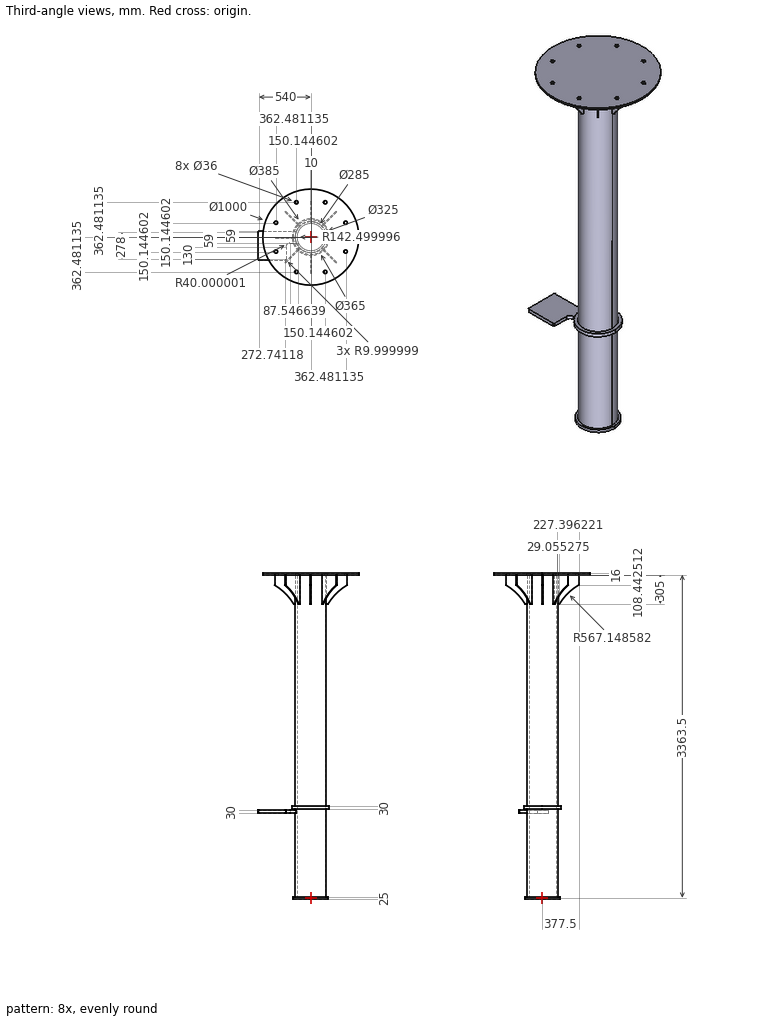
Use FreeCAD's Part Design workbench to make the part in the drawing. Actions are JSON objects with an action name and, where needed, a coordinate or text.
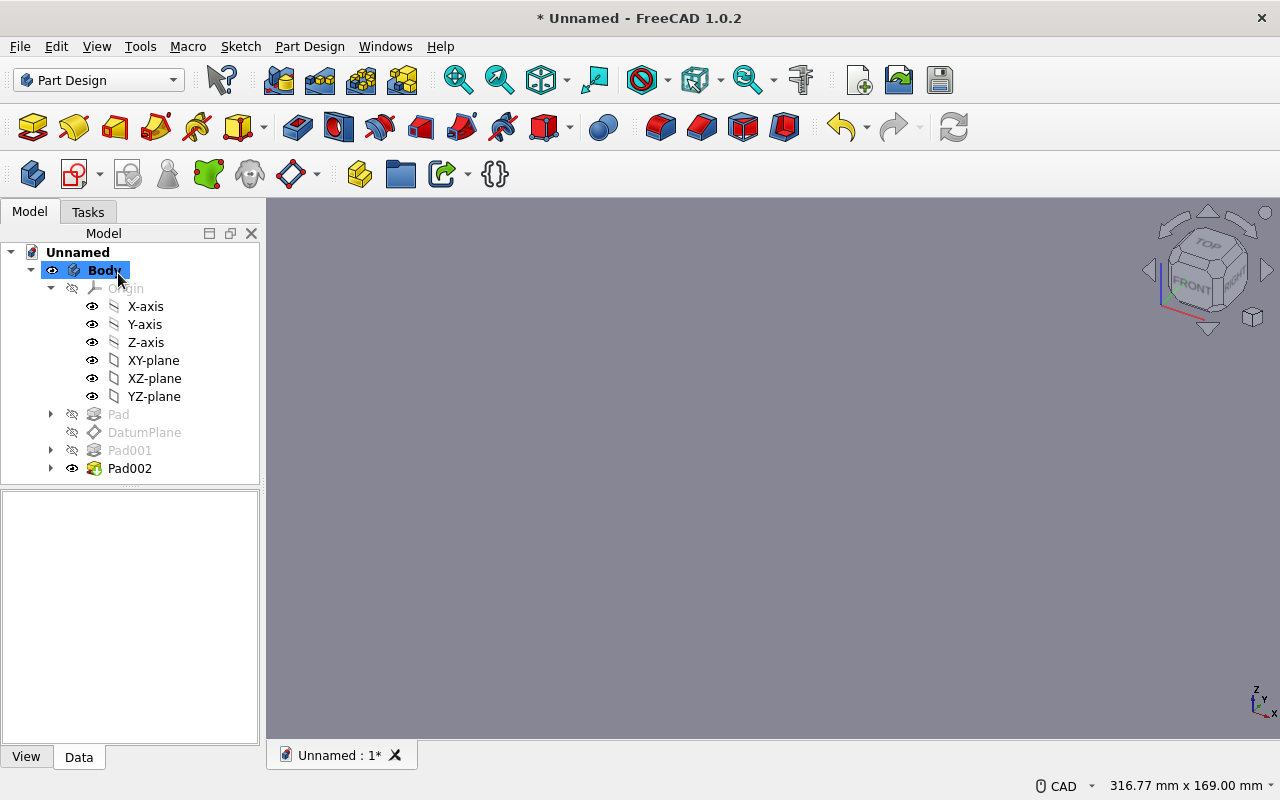
{"action": "key", "text": "v f"}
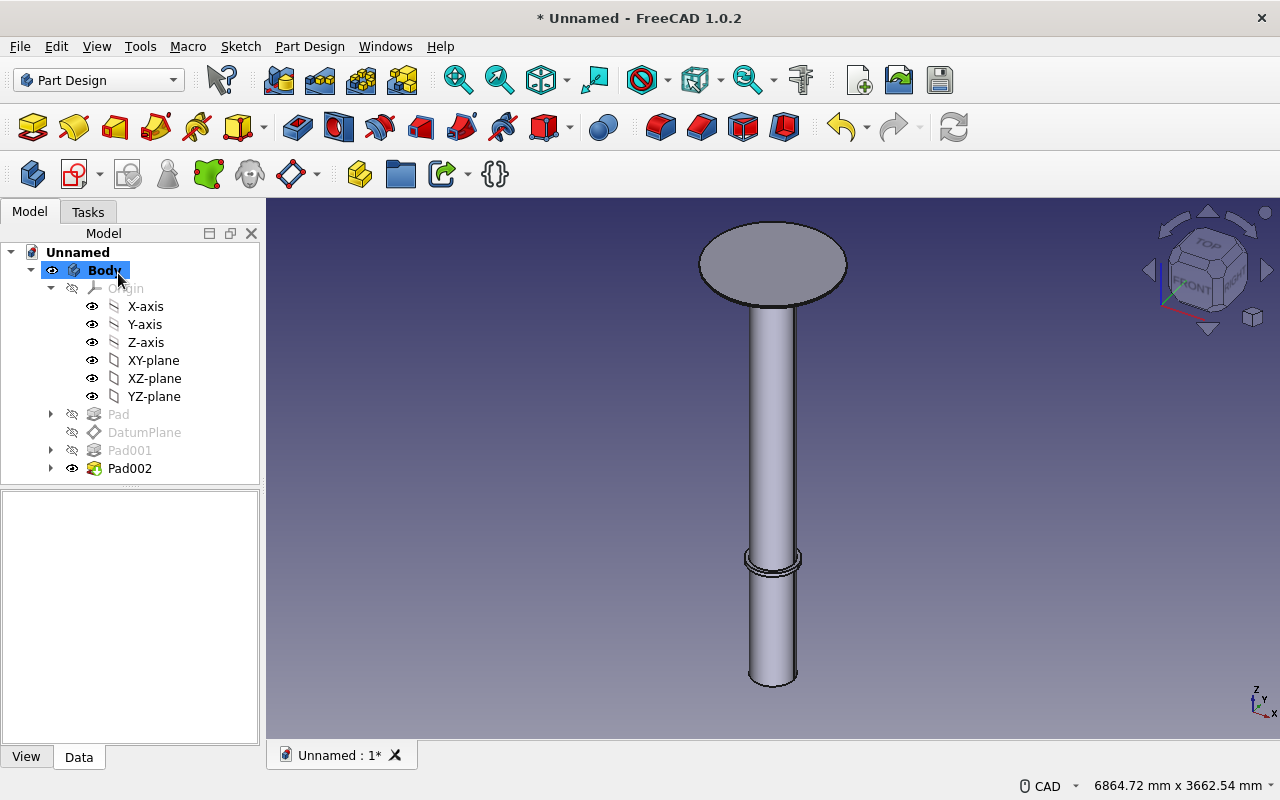
{"action": "left_click", "coordinate": [74, 174]}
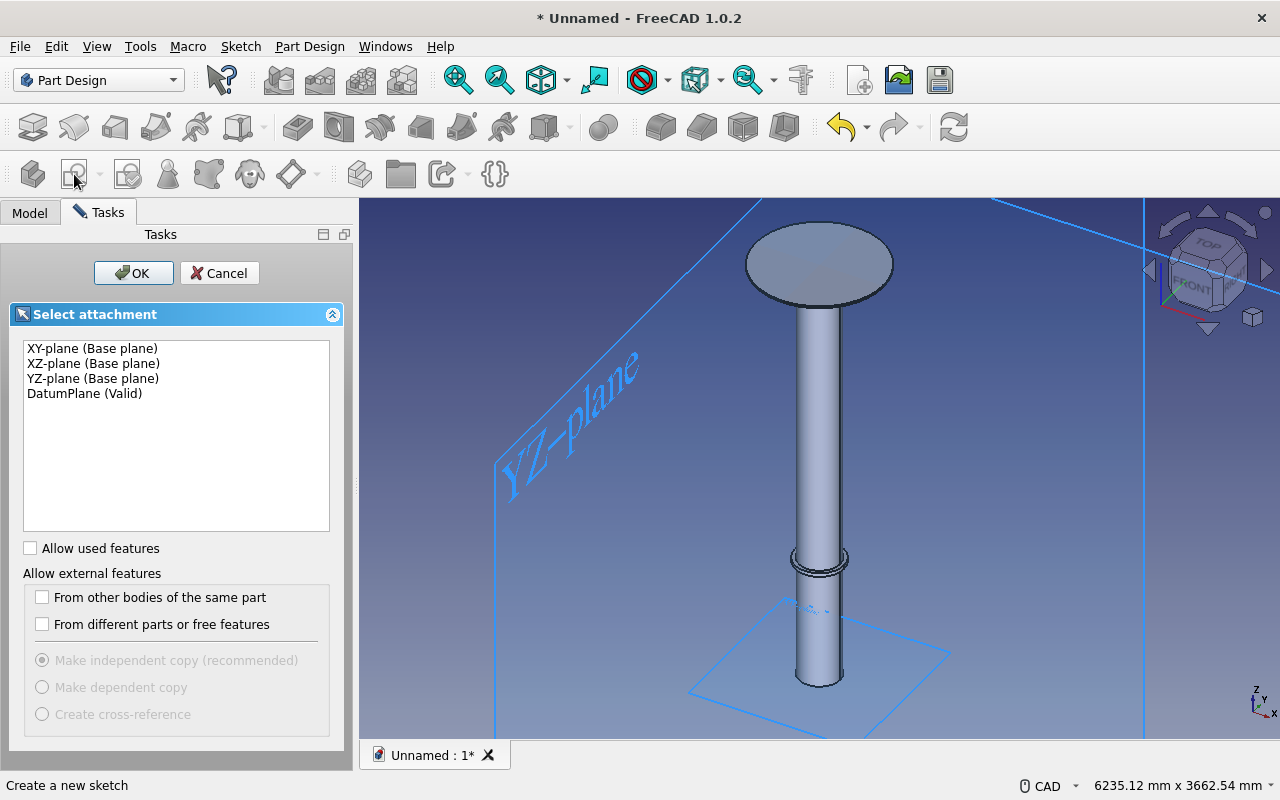
{"action": "left_click", "coordinate": [84, 378]}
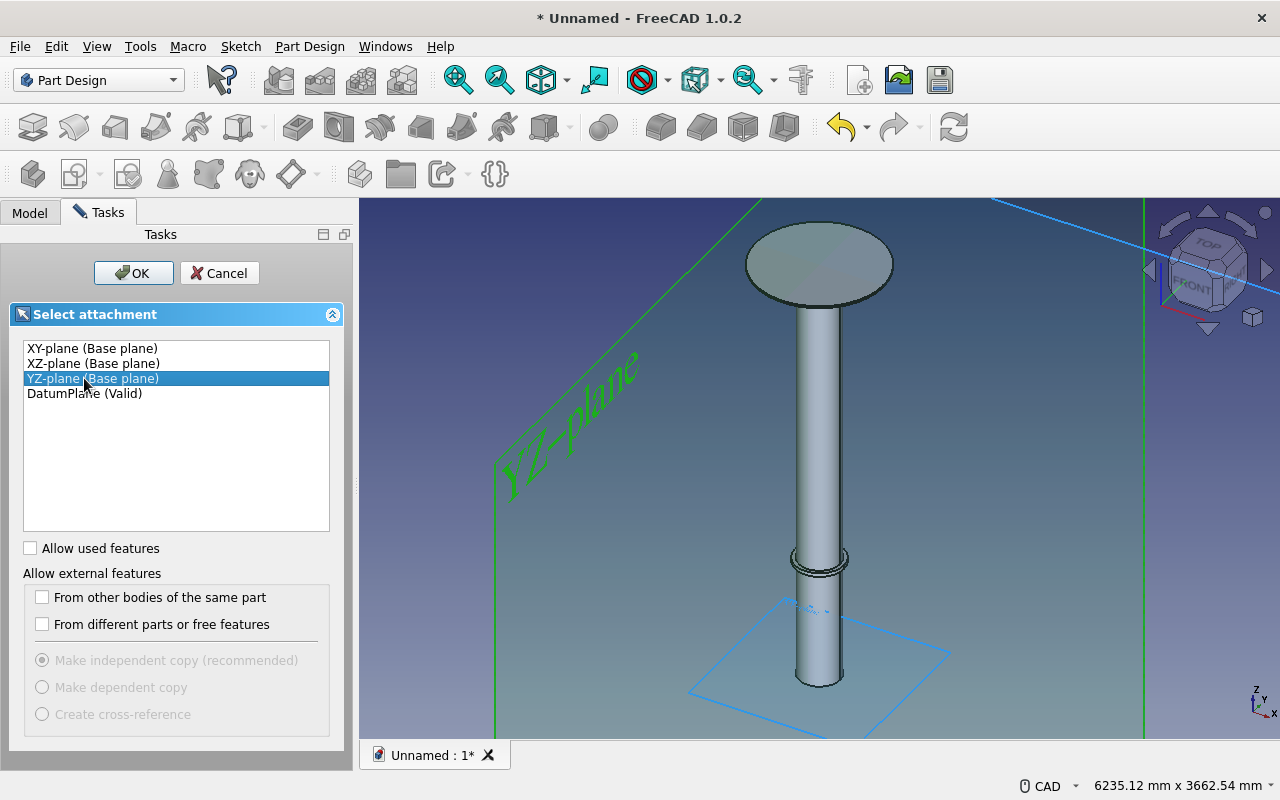
{"action": "left_click", "coordinate": [134, 273]}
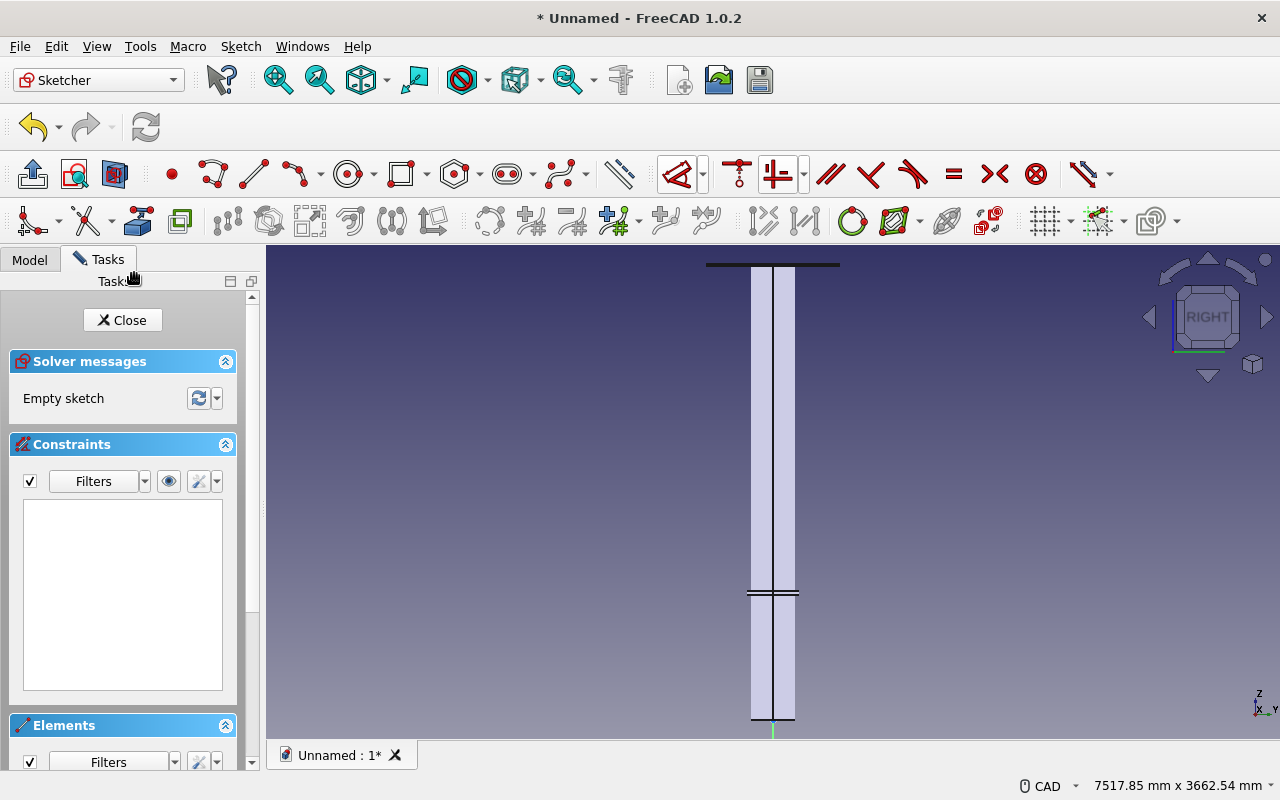
{"action": "key", "text": "q s"}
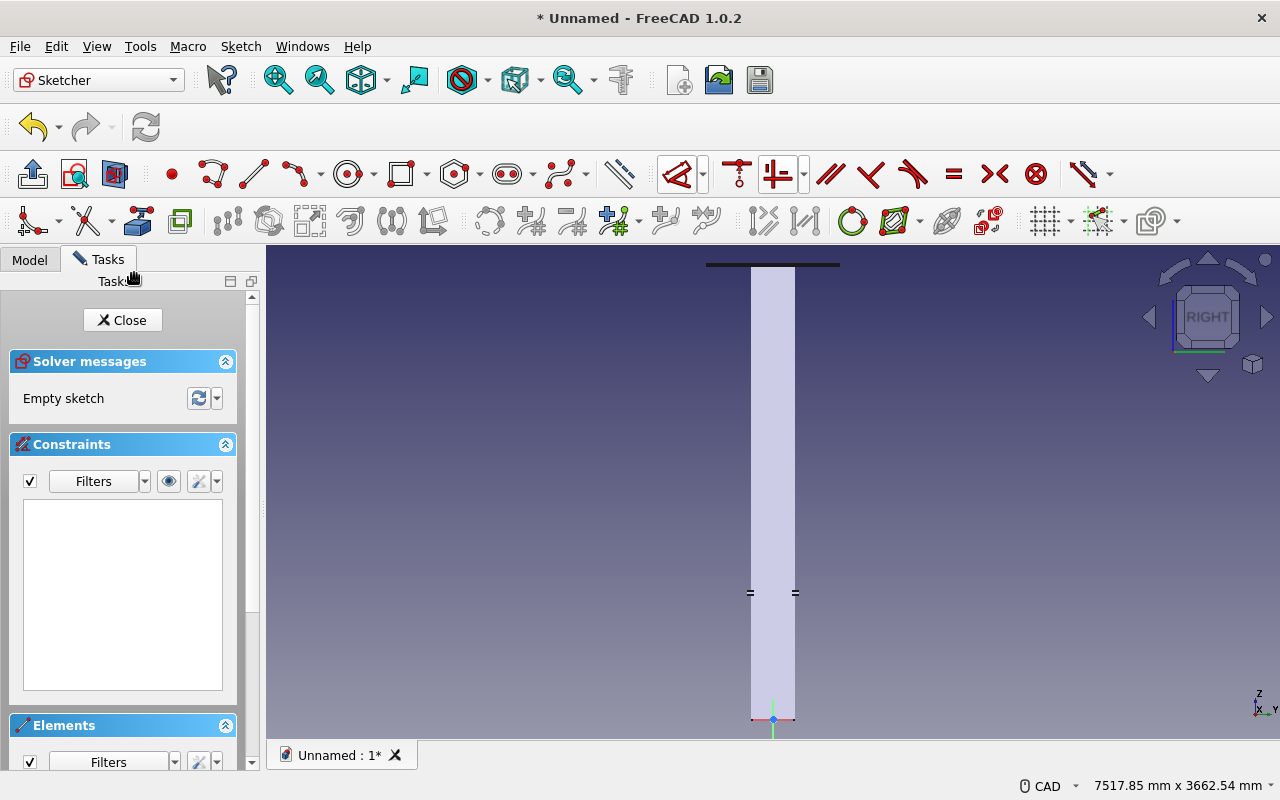
{"action": "scroll", "coordinate": [704, 492], "scroll_direction": "down", "scroll_amount": 5}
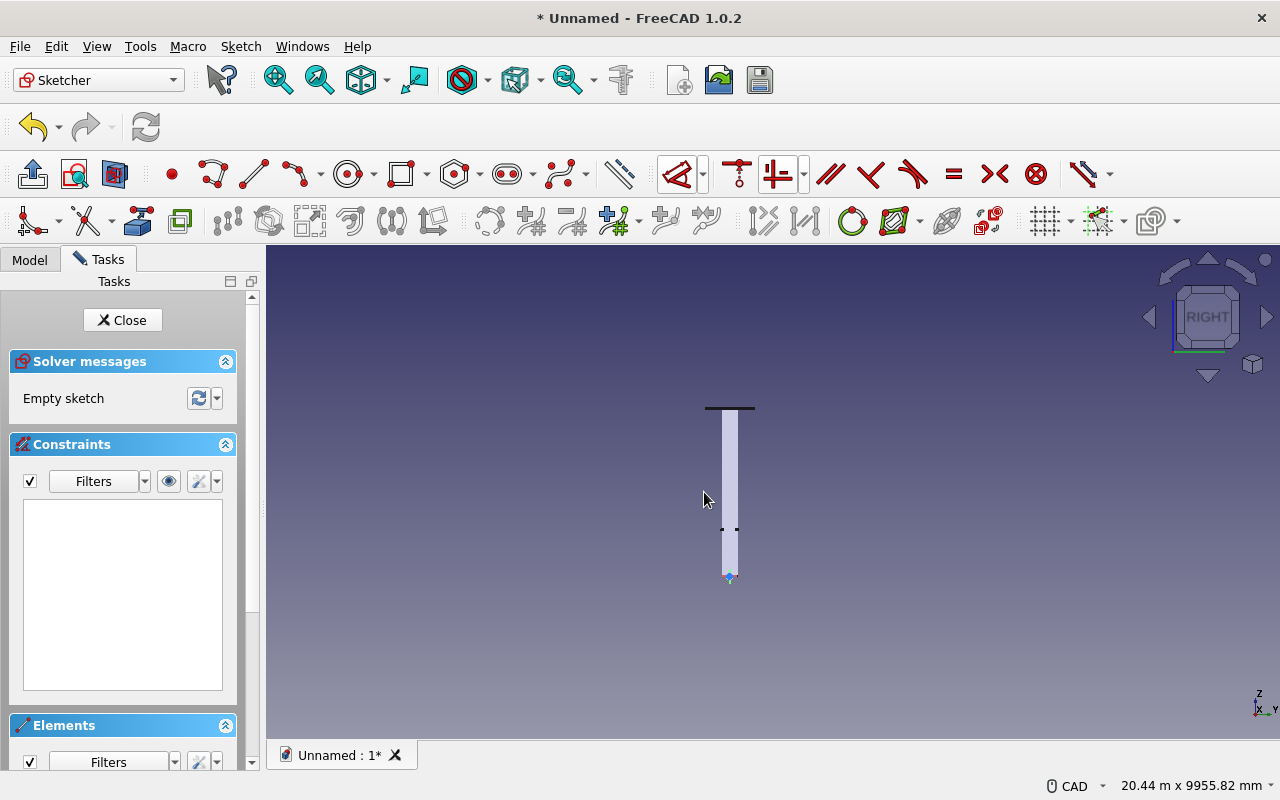
{"action": "scroll", "coordinate": [745, 413], "scroll_direction": "up", "scroll_amount": 15}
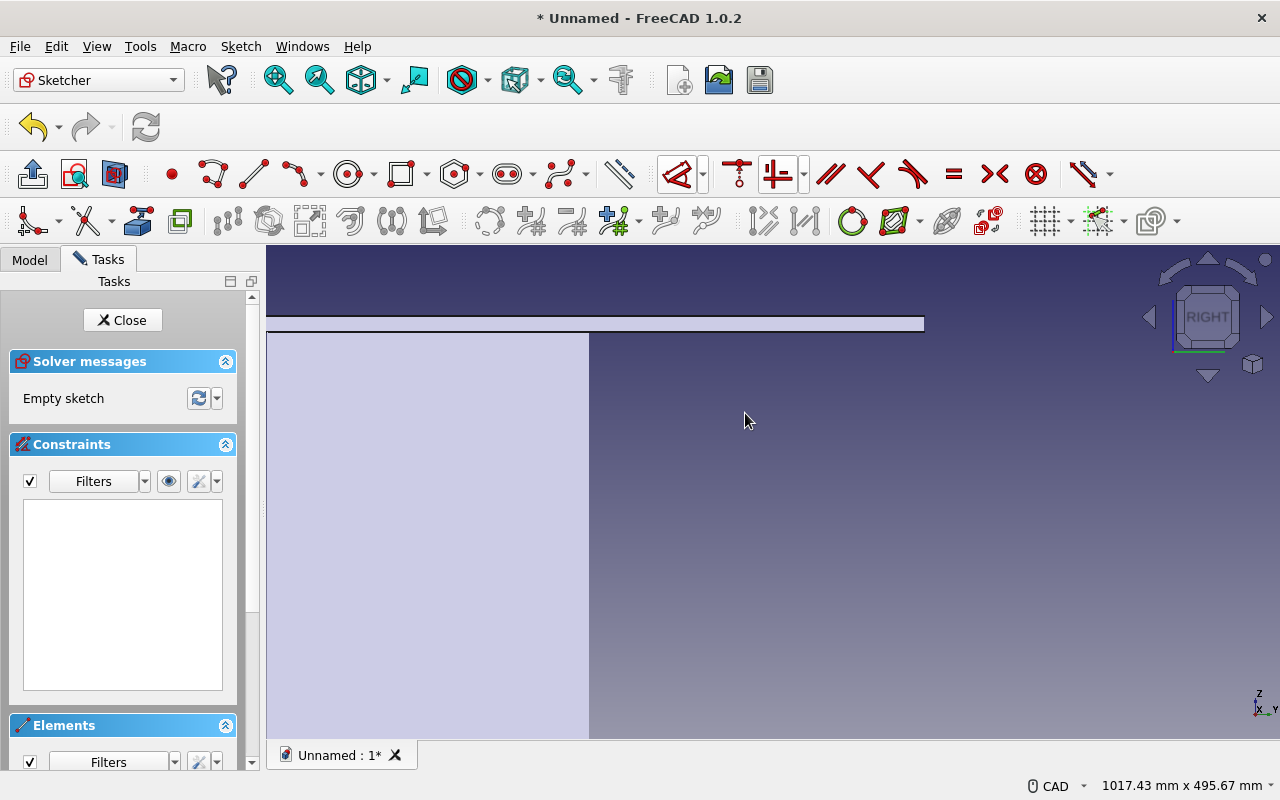
{"action": "key", "text": "g m"}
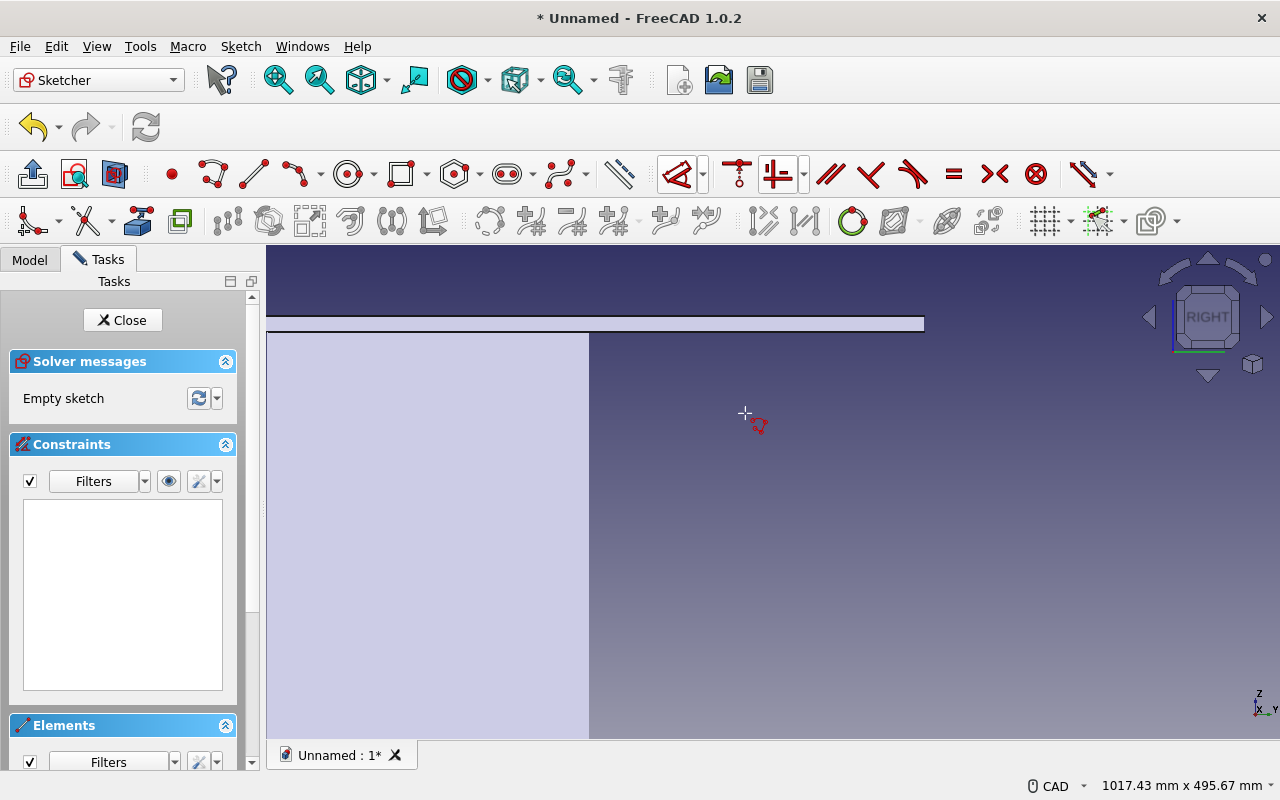
{"action": "left_click", "coordinate": [804, 440]}
{"action": "left_click", "coordinate": [804, 332]}
{"action": "left_click", "coordinate": [577, 332]}
{"action": "left_click", "coordinate": [577, 635]}
{"action": "left_click", "coordinate": [606, 635]}
{"action": "right_click", "coordinate": [606, 635]}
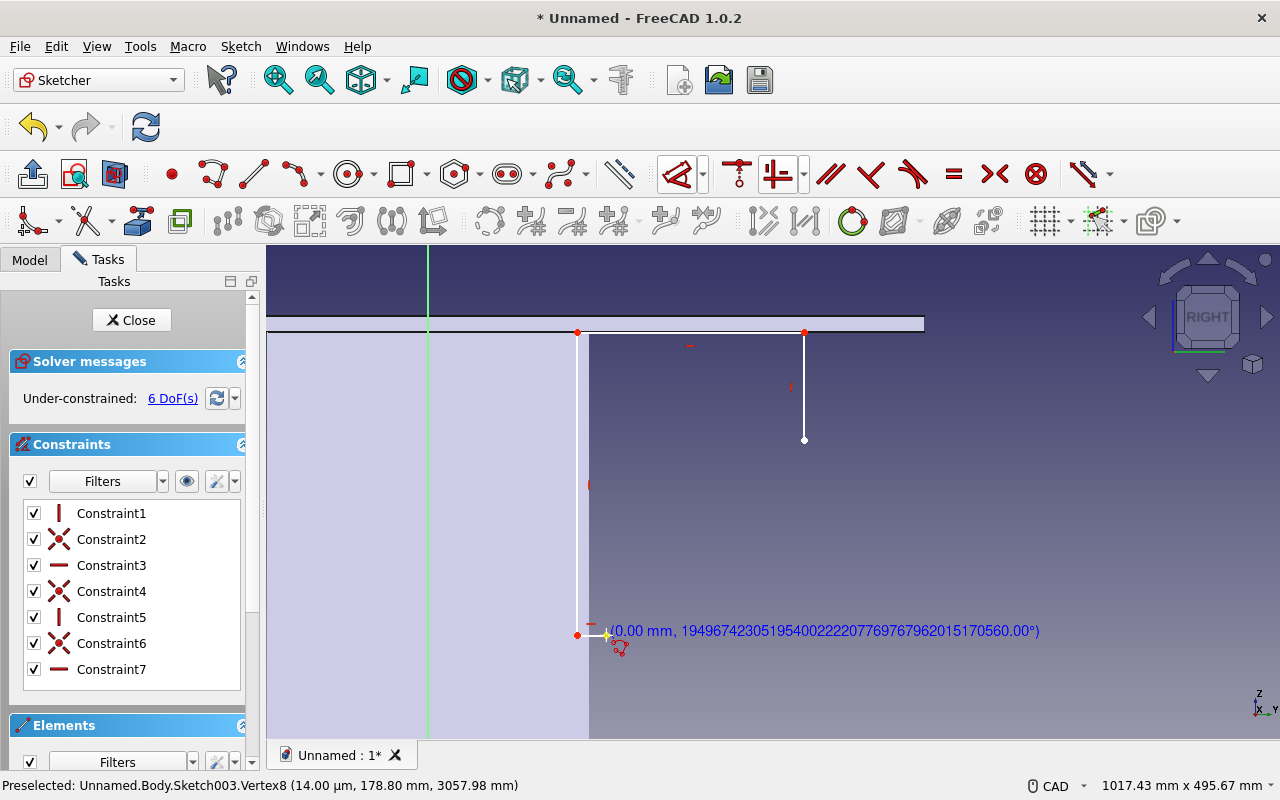
{"action": "left_click", "coordinate": [294, 174]}